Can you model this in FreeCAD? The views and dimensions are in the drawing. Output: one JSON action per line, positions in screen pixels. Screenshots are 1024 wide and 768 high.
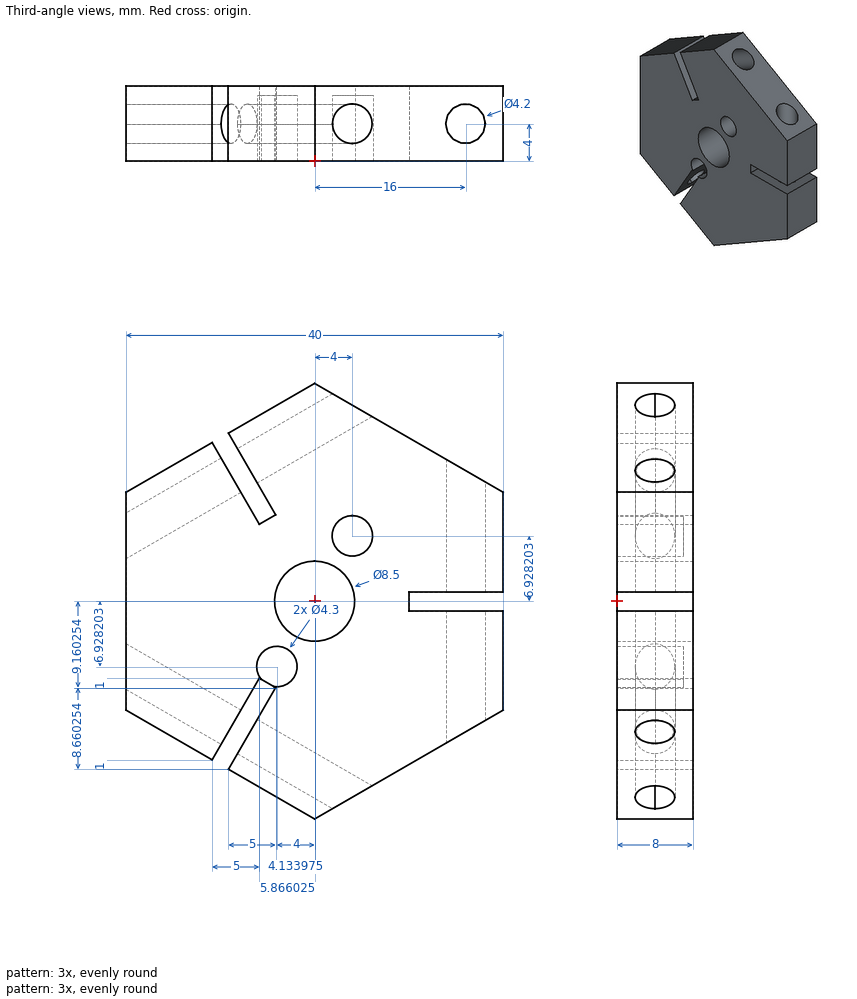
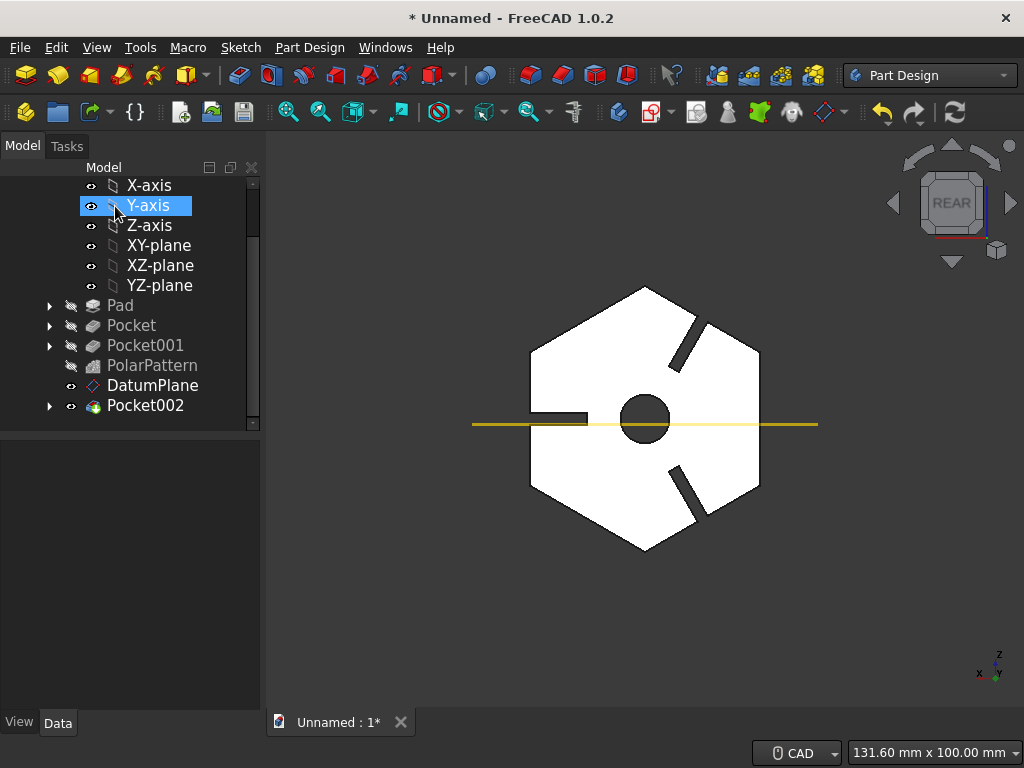
{"action": "left_click", "coordinate": [116, 386]}
{"action": "key", "text": "space"}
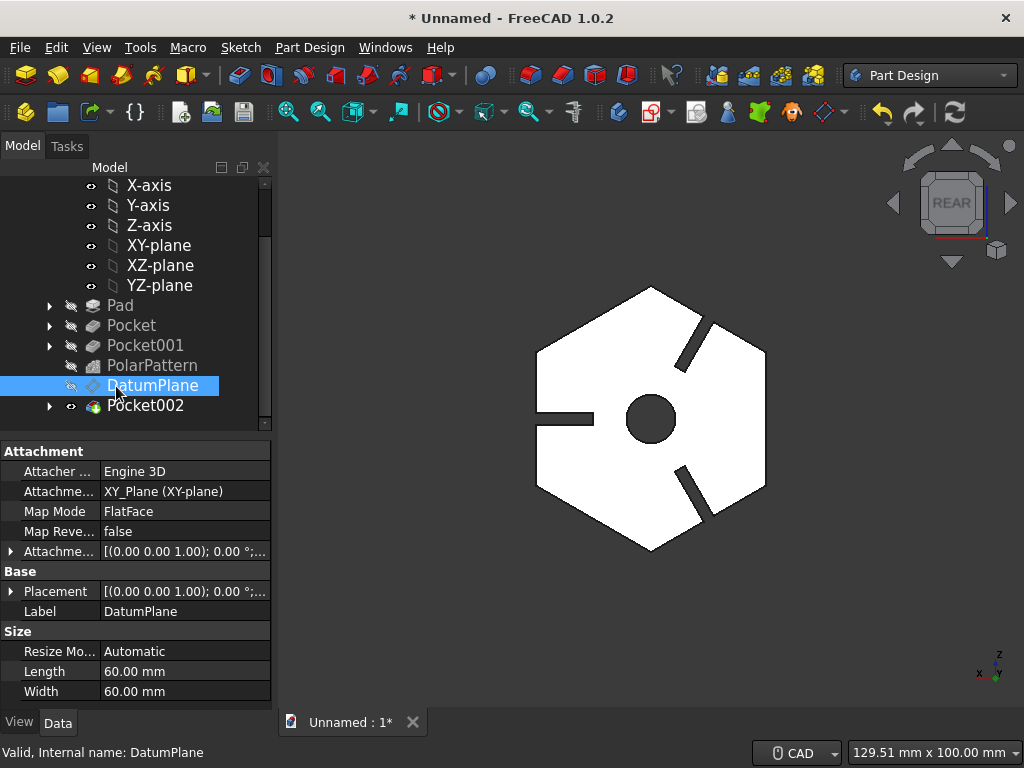
{"action": "left_click", "coordinate": [116, 406]}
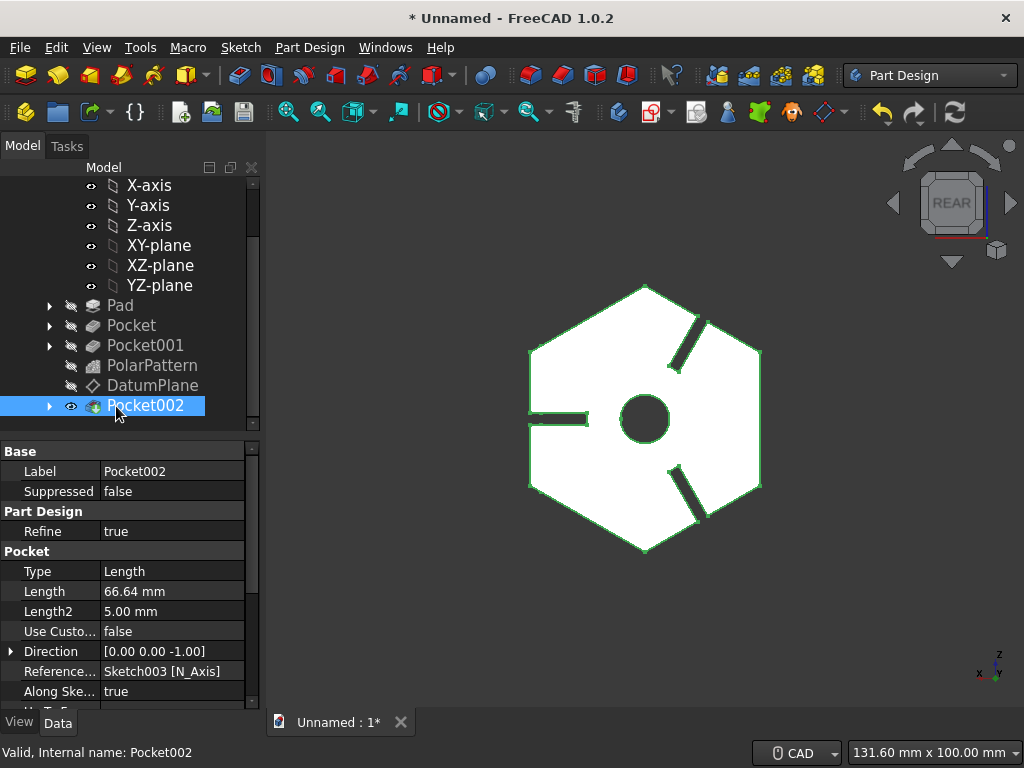
{"action": "left_click", "coordinate": [782, 76]}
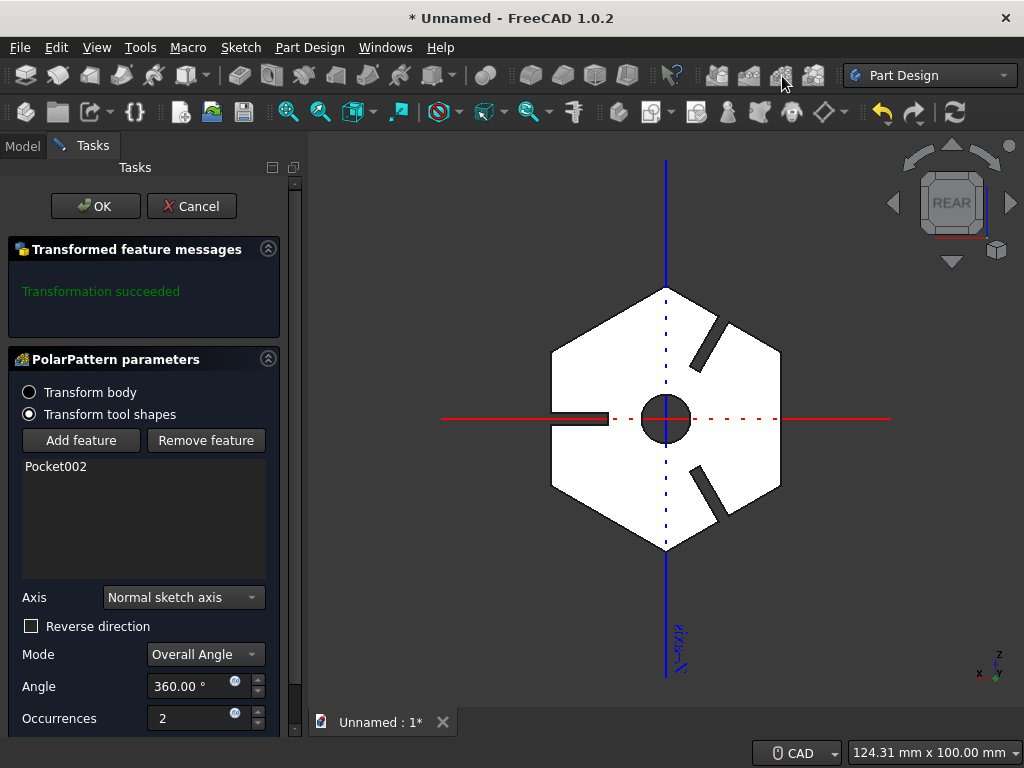
{"action": "left_click", "coordinate": [184, 598]}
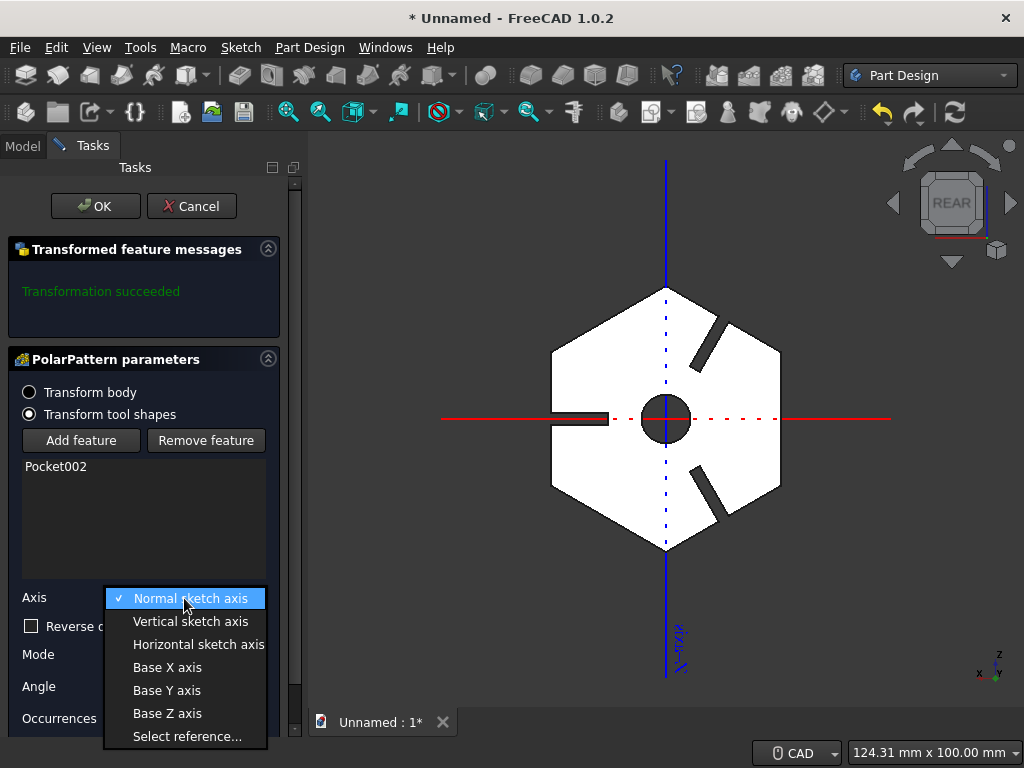
{"action": "left_click", "coordinate": [184, 690]}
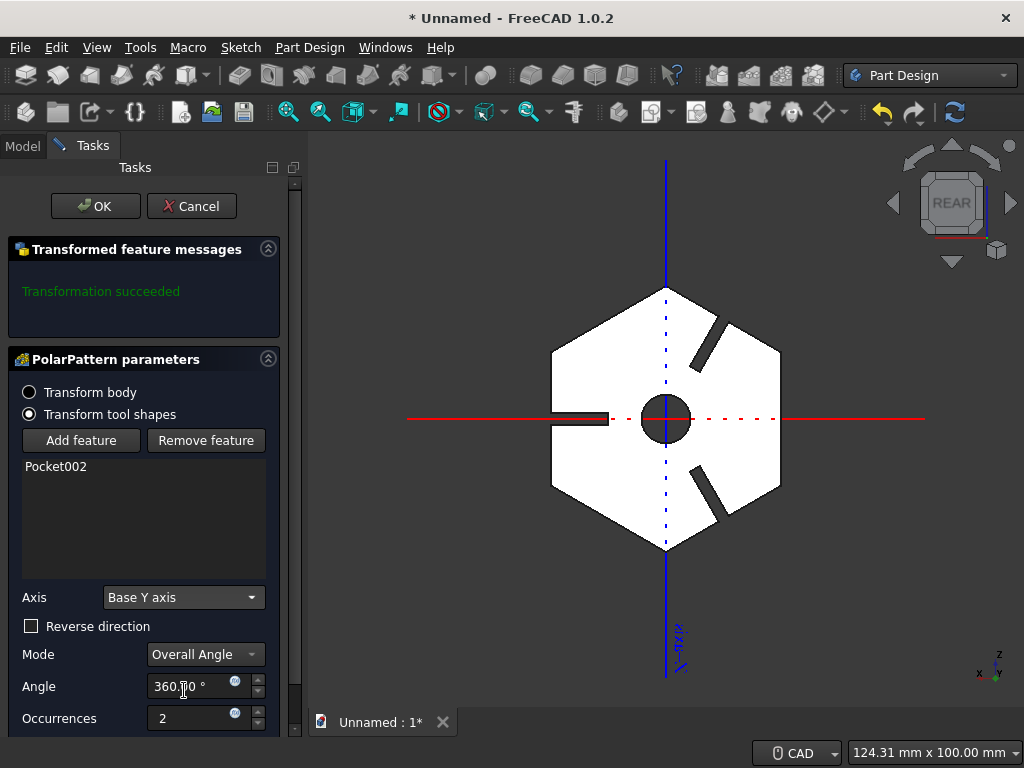
{"action": "triple_click", "coordinate": [198, 718]}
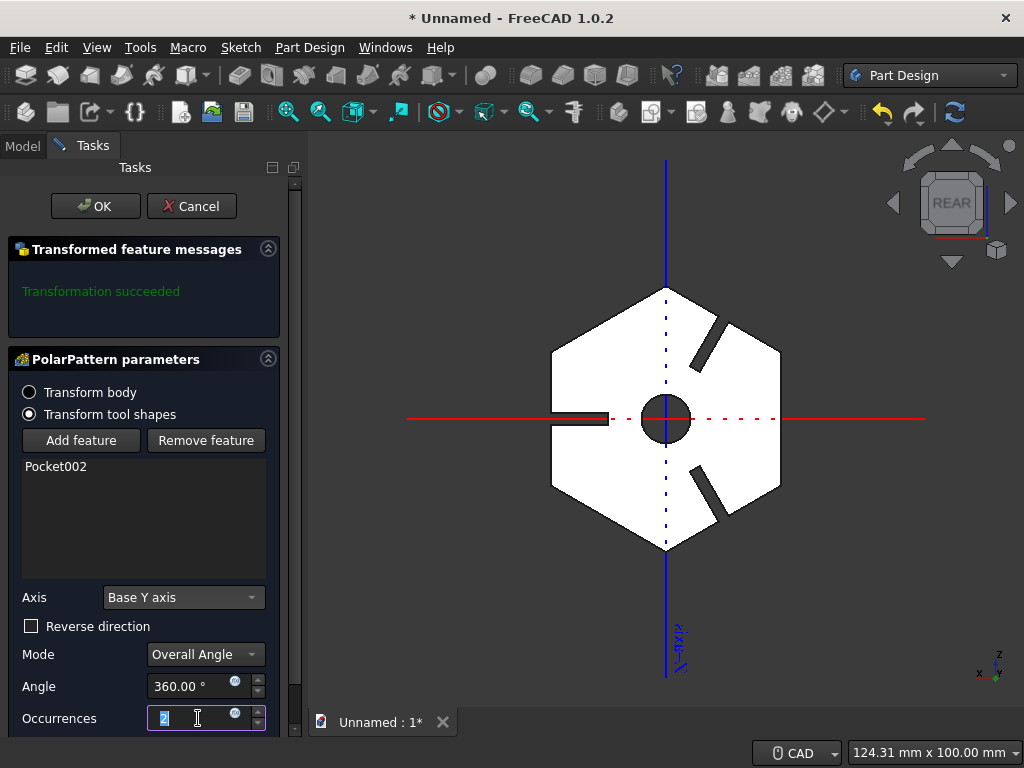
{"action": "type", "text": "3"}
{"action": "key", "text": "Tab"}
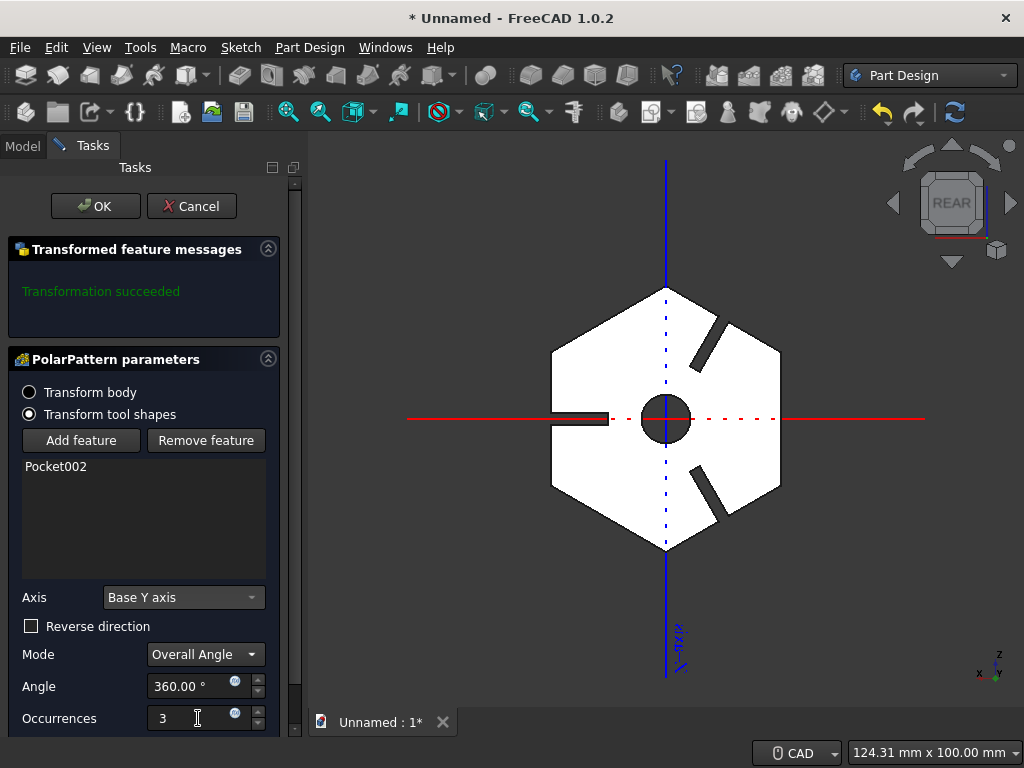
{"action": "left_click", "coordinate": [96, 206]}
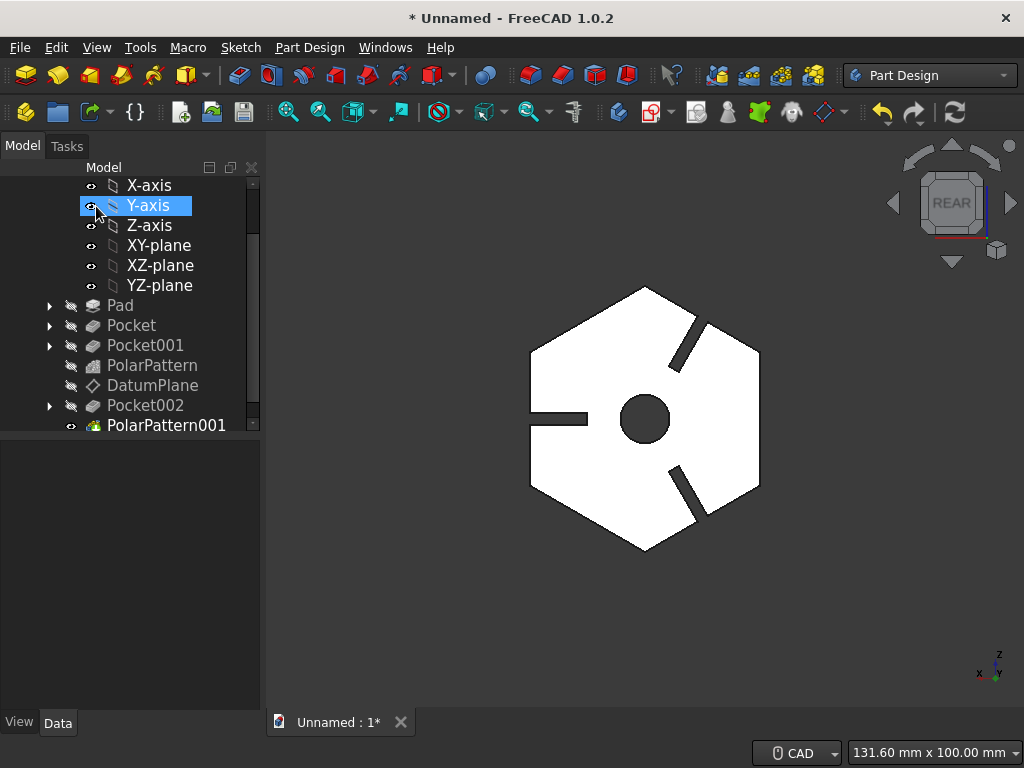
{"action": "scroll", "coordinate": [160, 301], "scroll_direction": "down", "scroll_amount": 3}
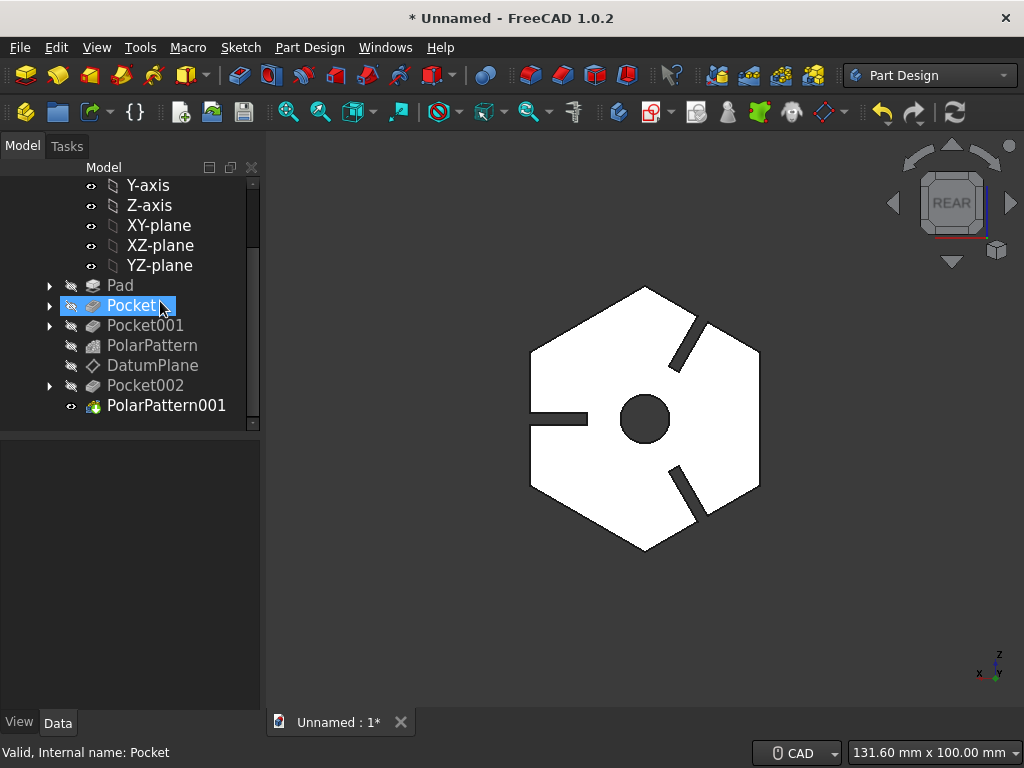
{"action": "scroll", "coordinate": [160, 301], "scroll_direction": "up", "scroll_amount": 15}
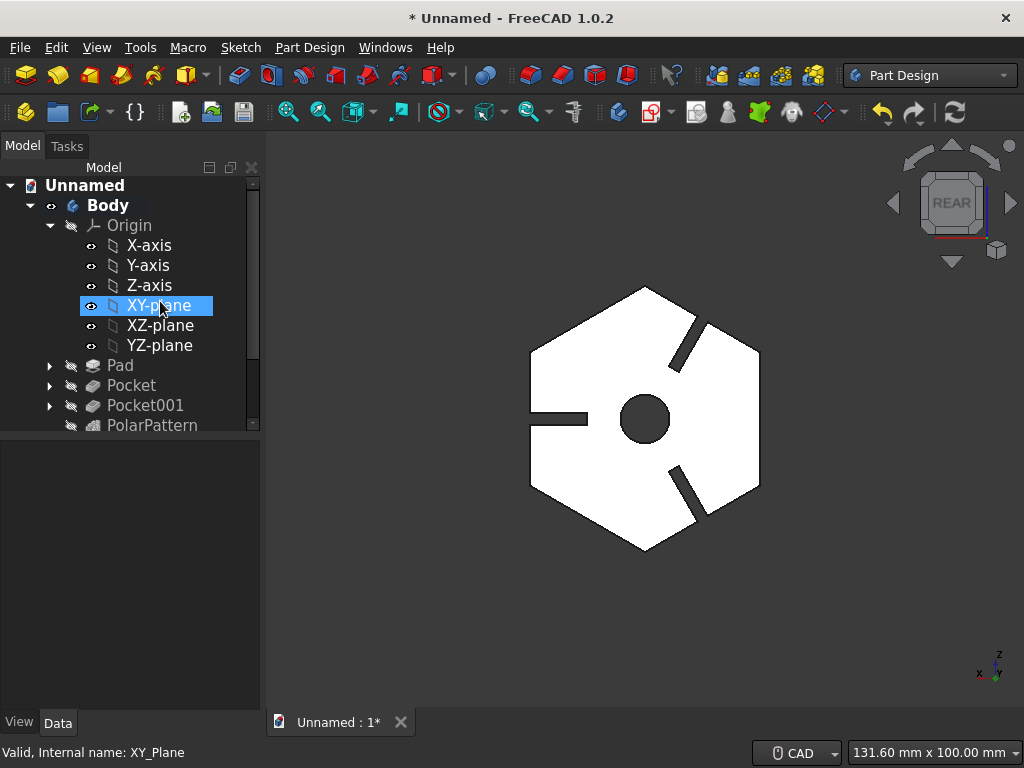
{"action": "left_click", "coordinate": [136, 326]}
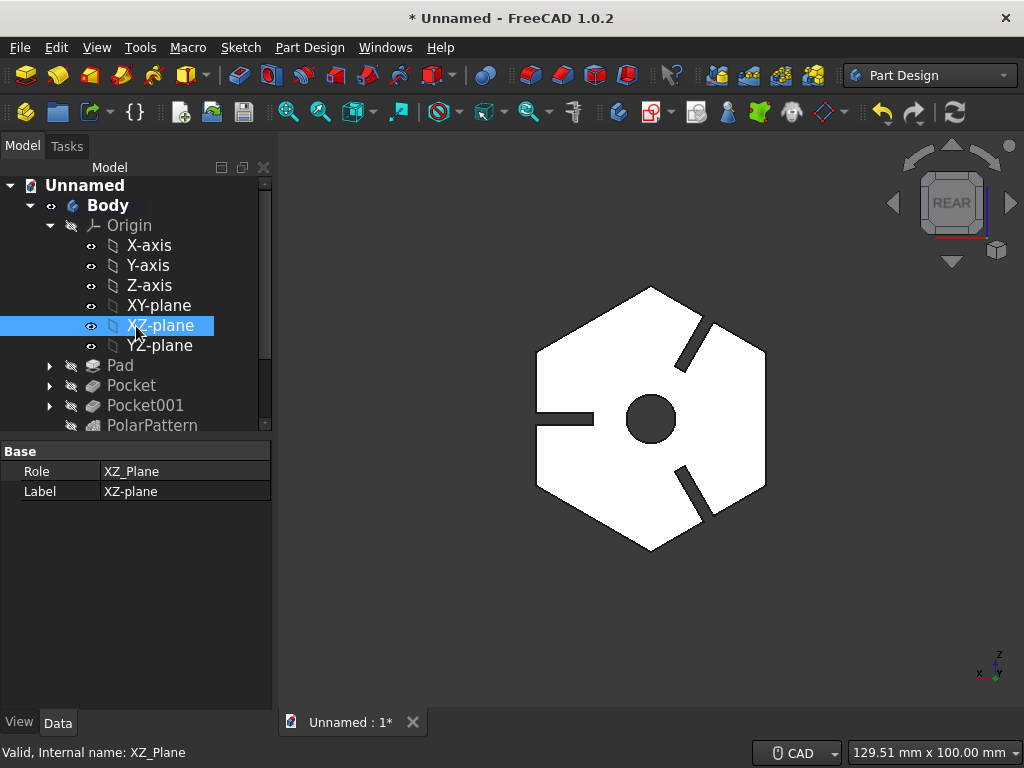
{"action": "left_click", "coordinate": [824, 112]}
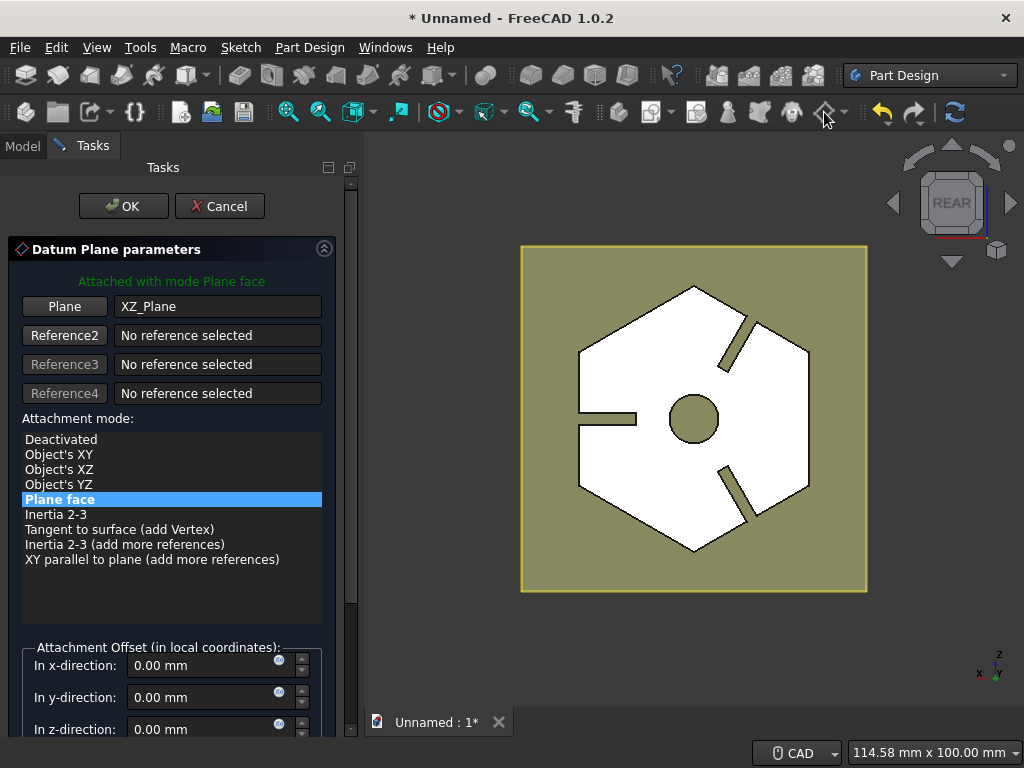
{"action": "scroll", "coordinate": [351, 456], "scroll_direction": "down", "scroll_amount": 2}